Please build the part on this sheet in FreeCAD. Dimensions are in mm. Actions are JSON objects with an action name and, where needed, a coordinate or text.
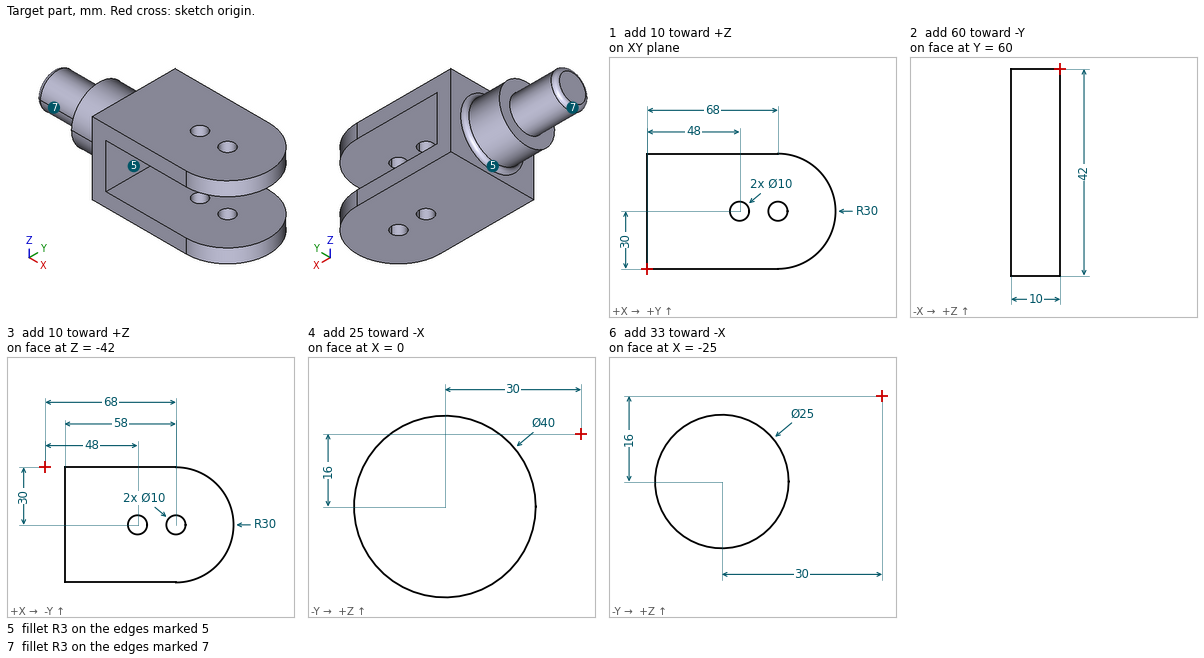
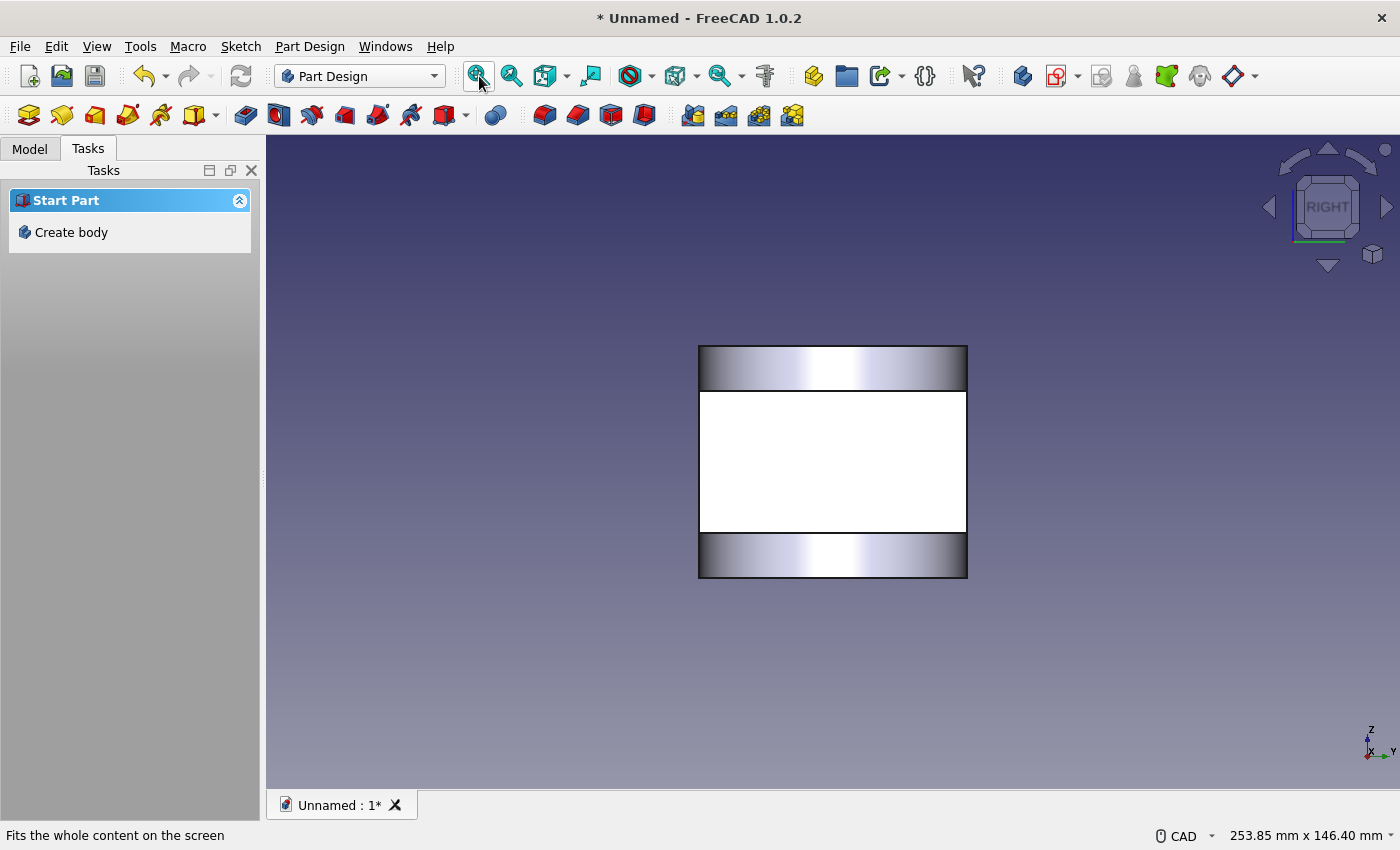
{"action": "key", "text": "5"}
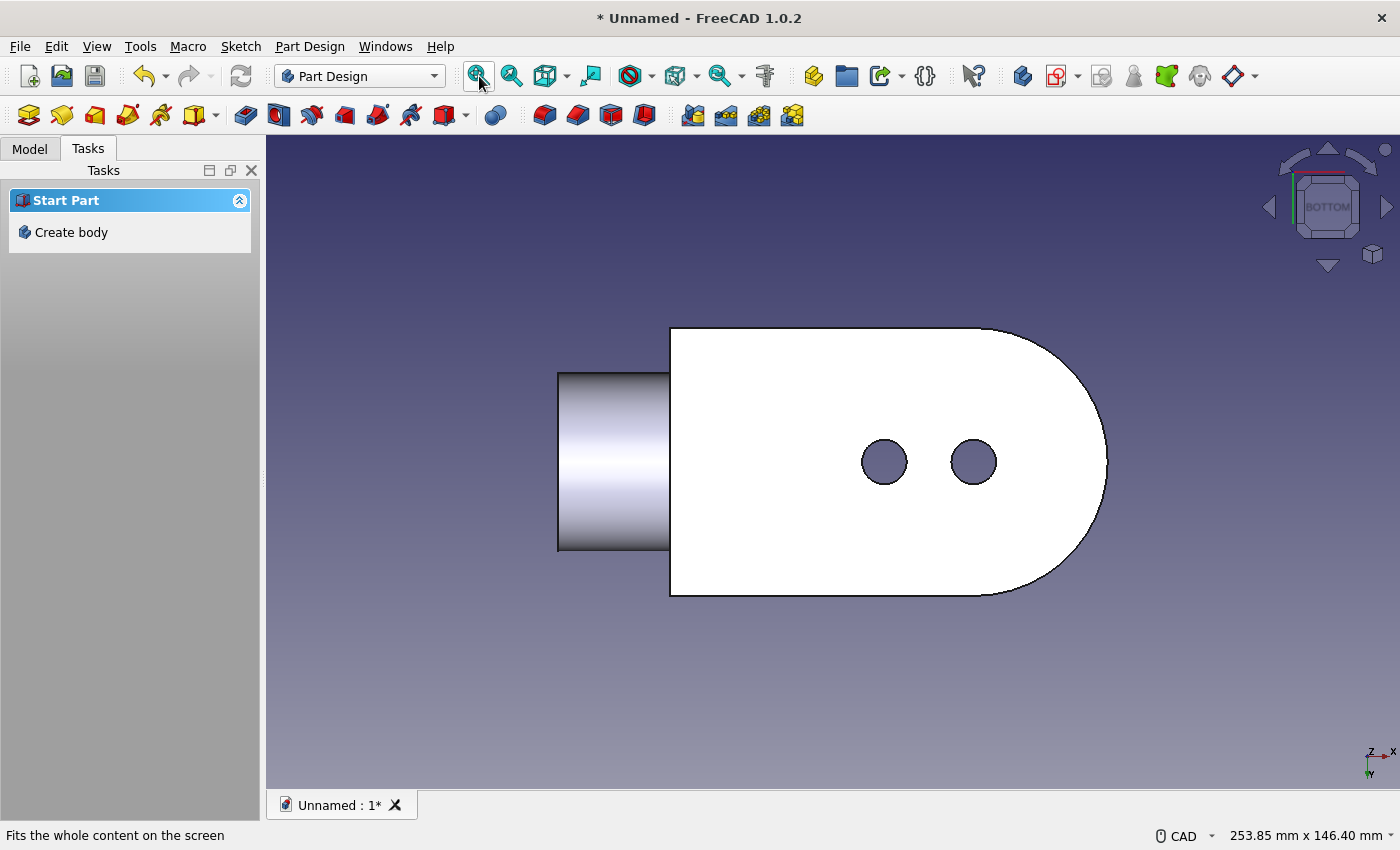
{"action": "key", "text": "4"}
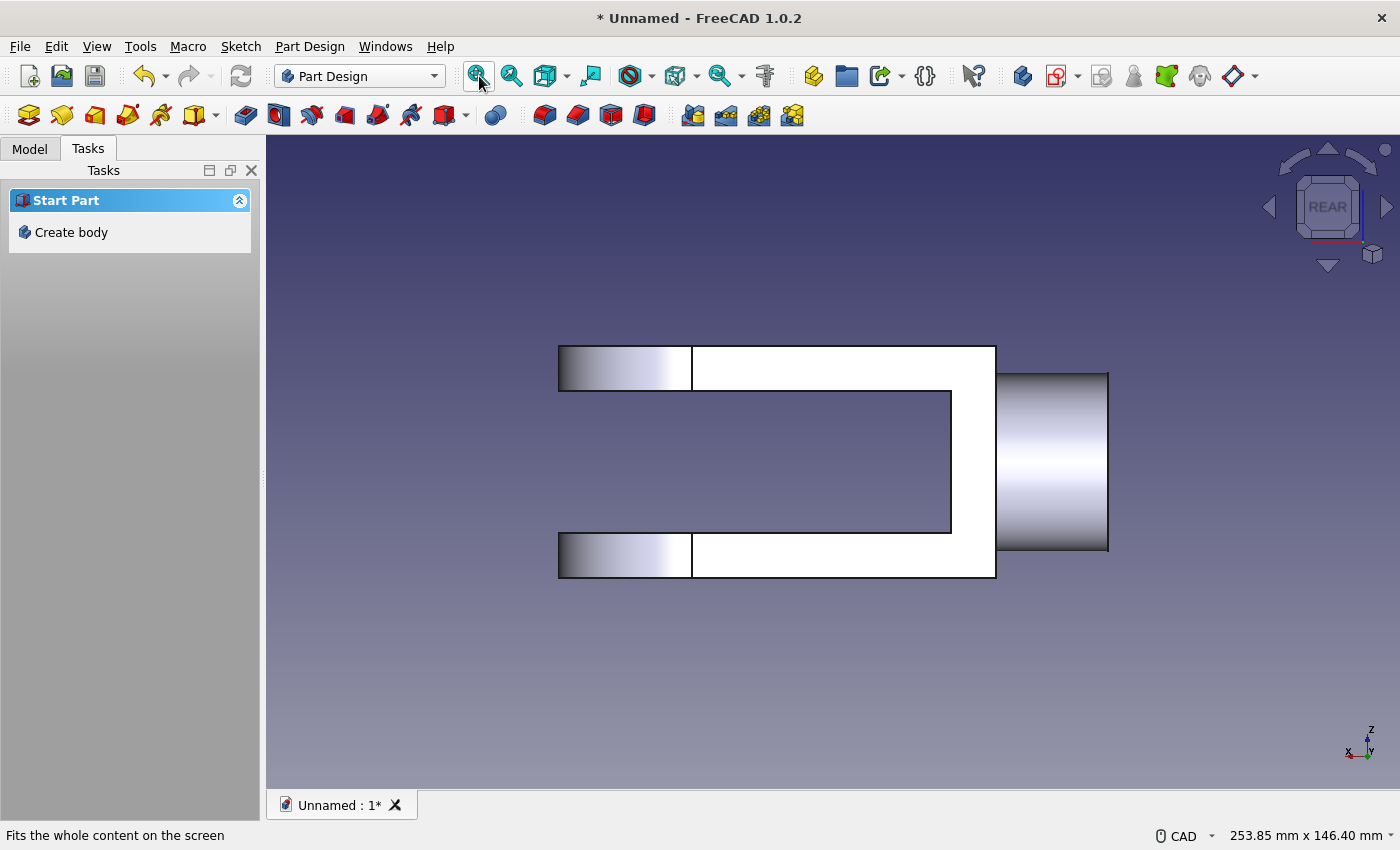
{"action": "key", "text": "6"}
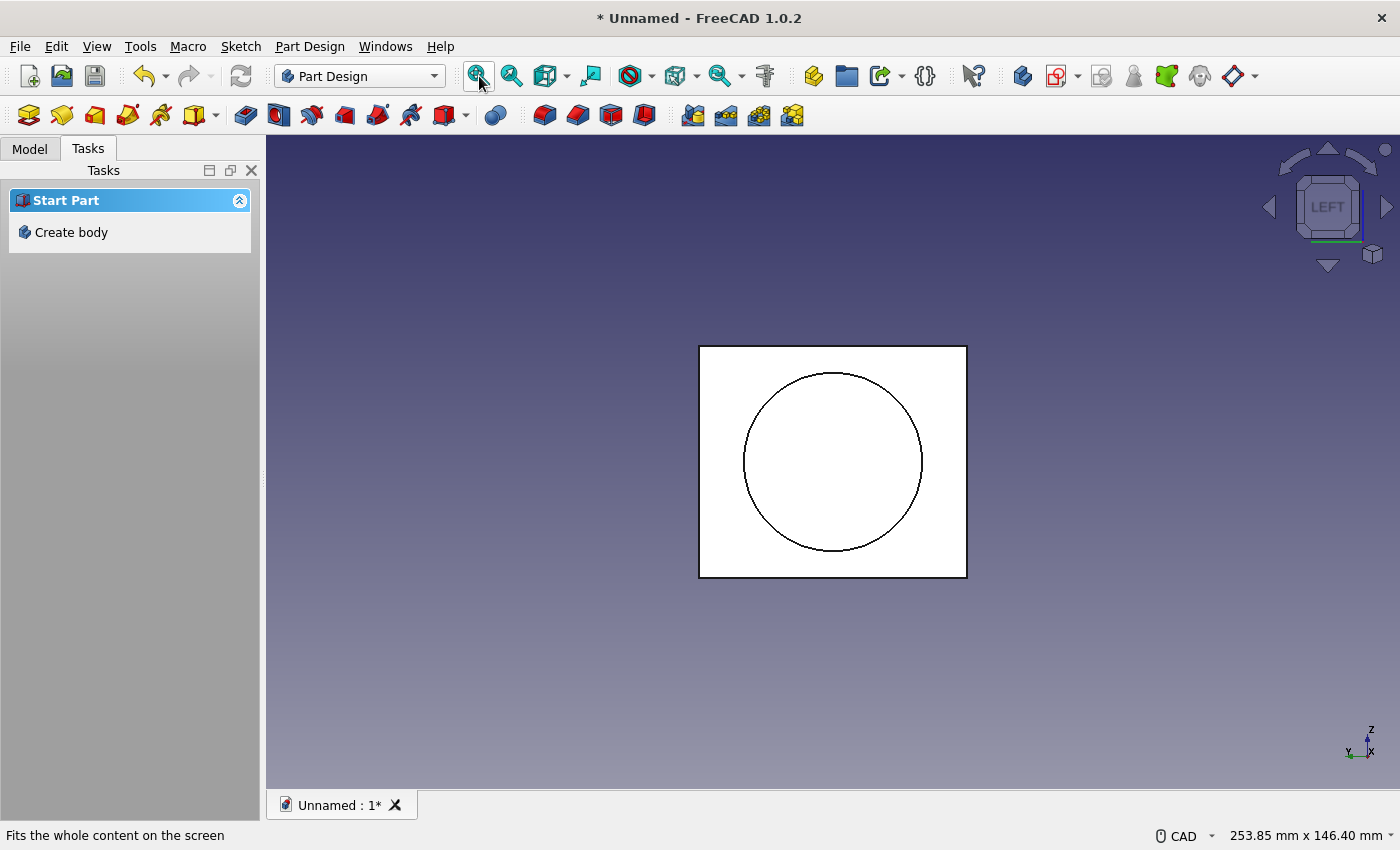
{"action": "key", "text": "v f"}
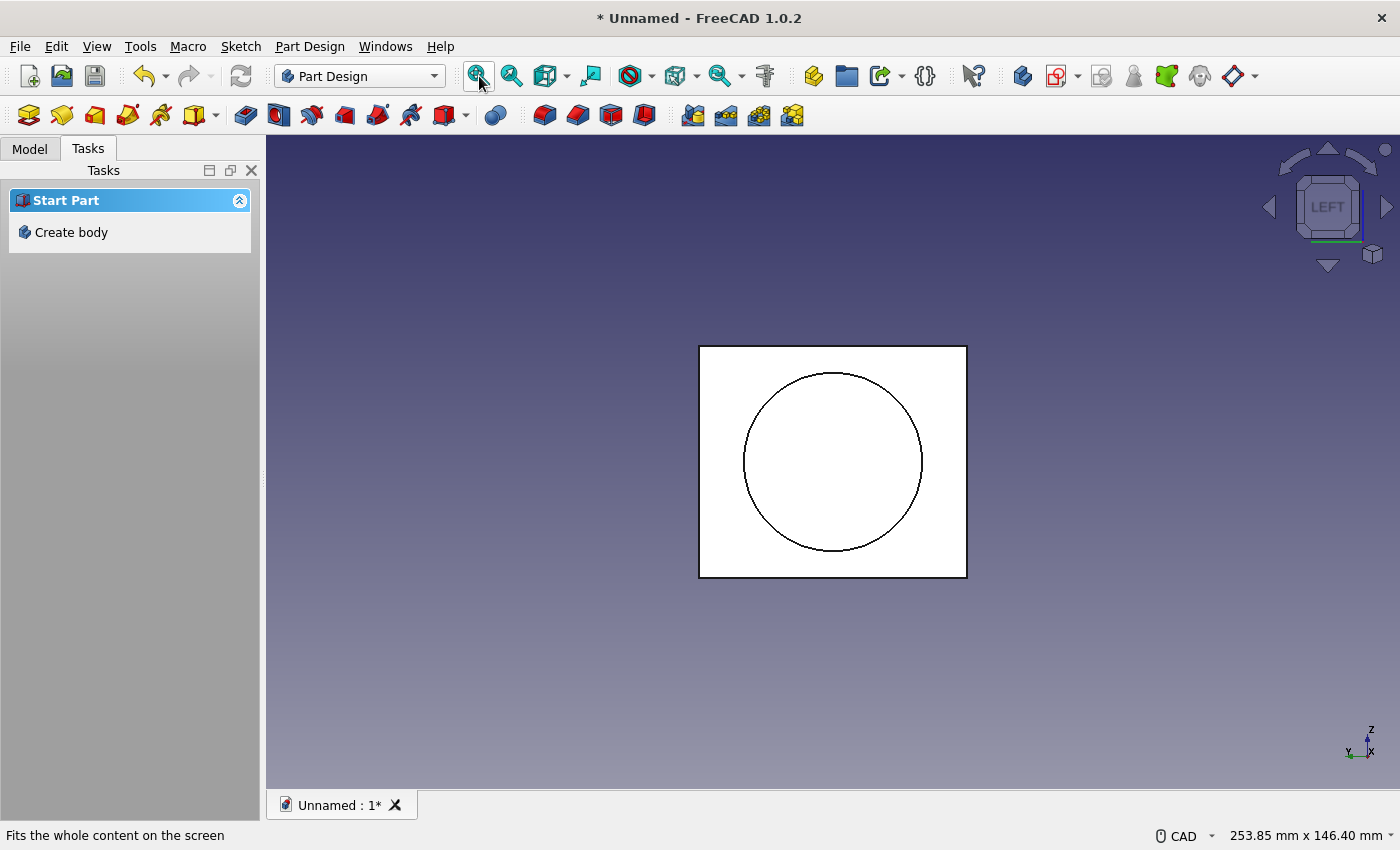
{"action": "key", "text": "v 3"}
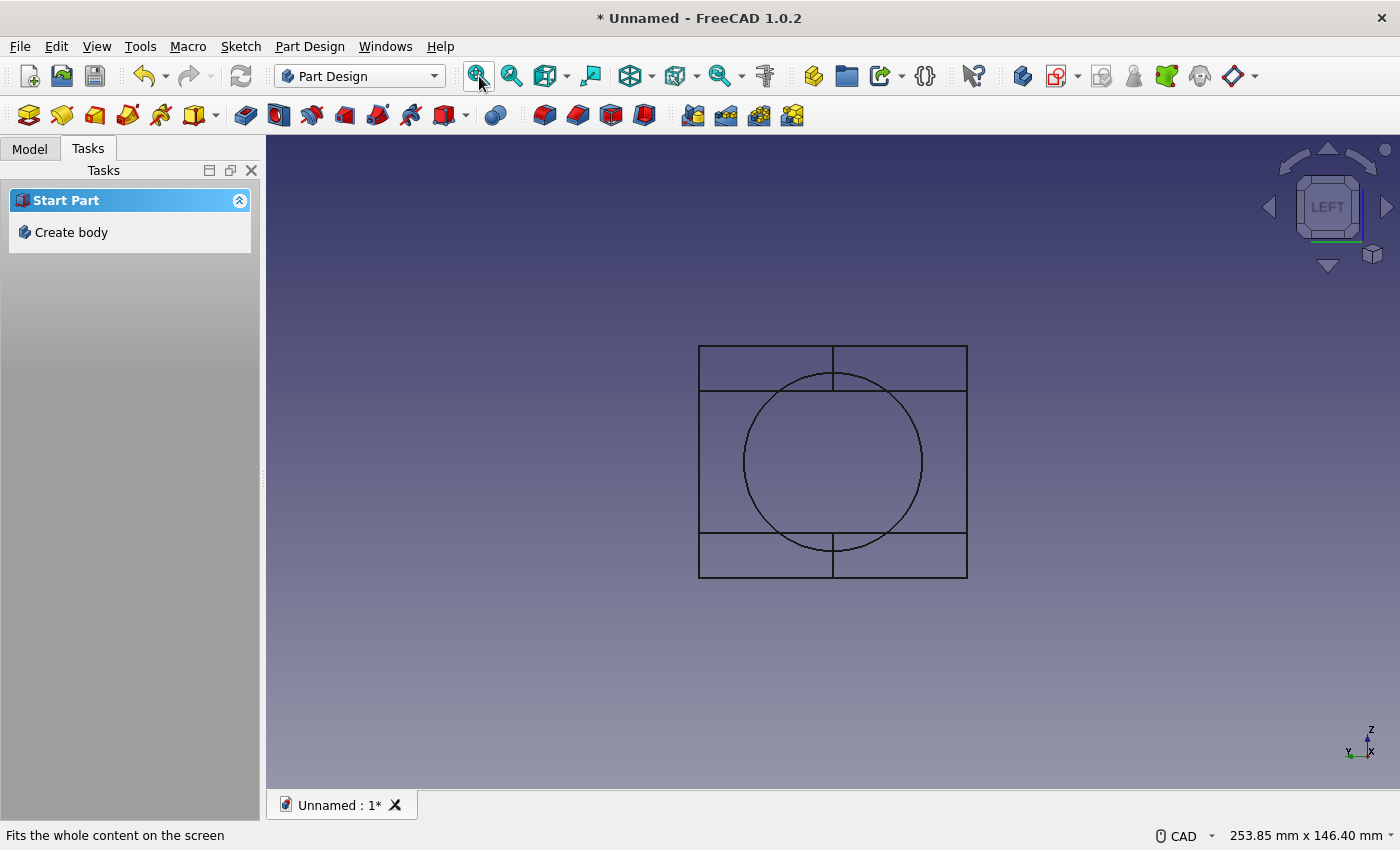
{"action": "key", "text": "0"}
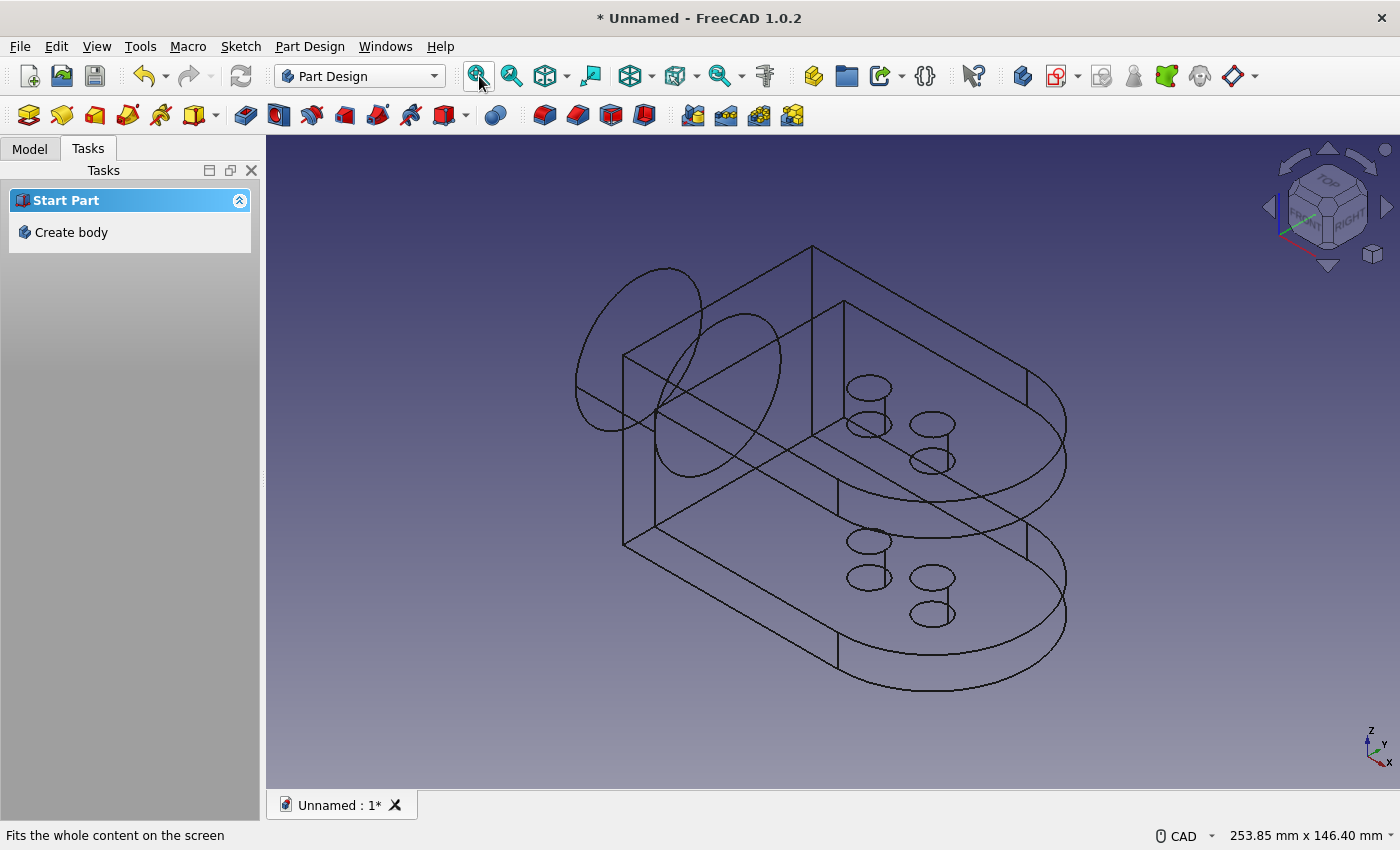
{"action": "left_click", "coordinate": [781, 358]}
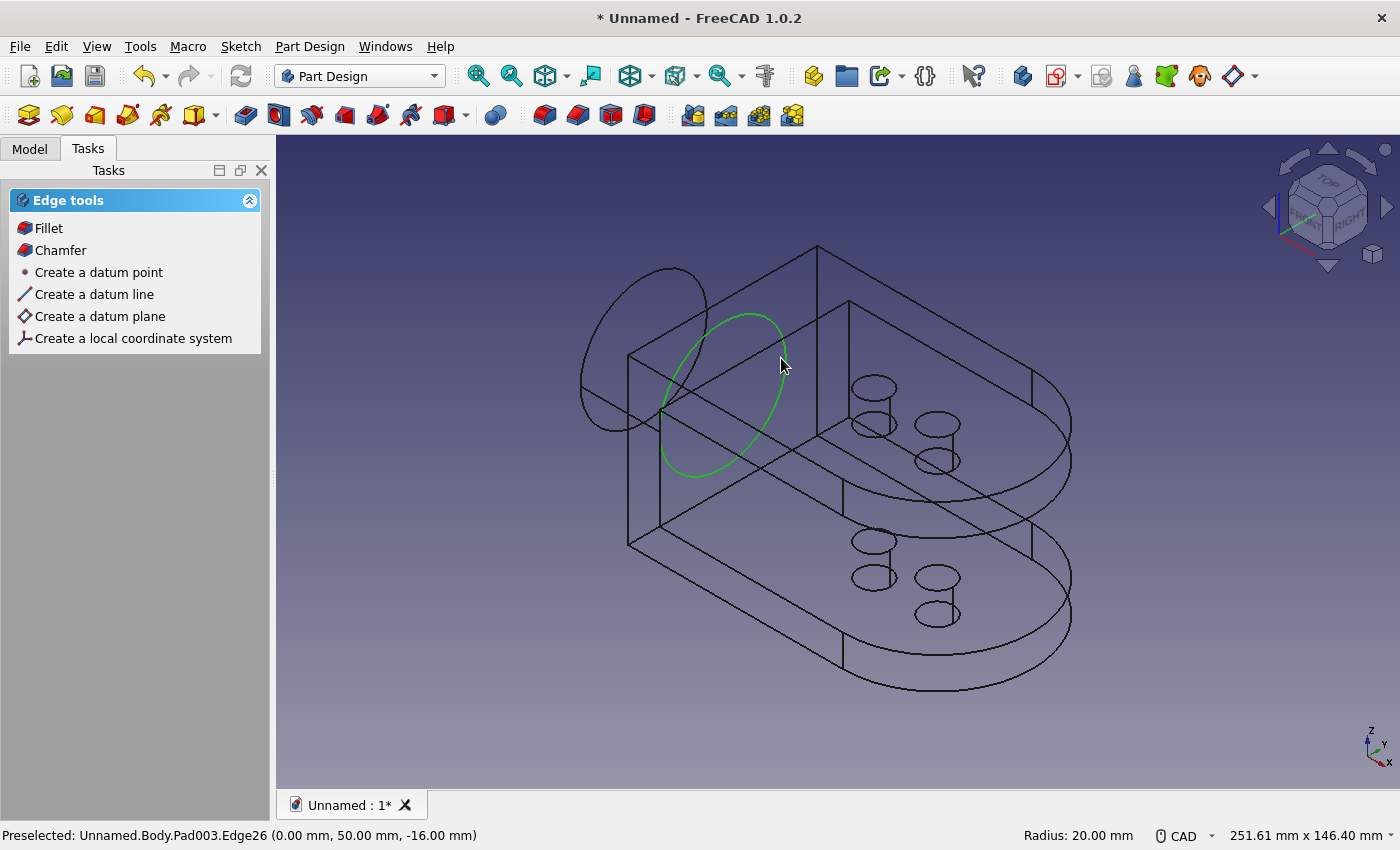
{"action": "key", "text": "v 1"}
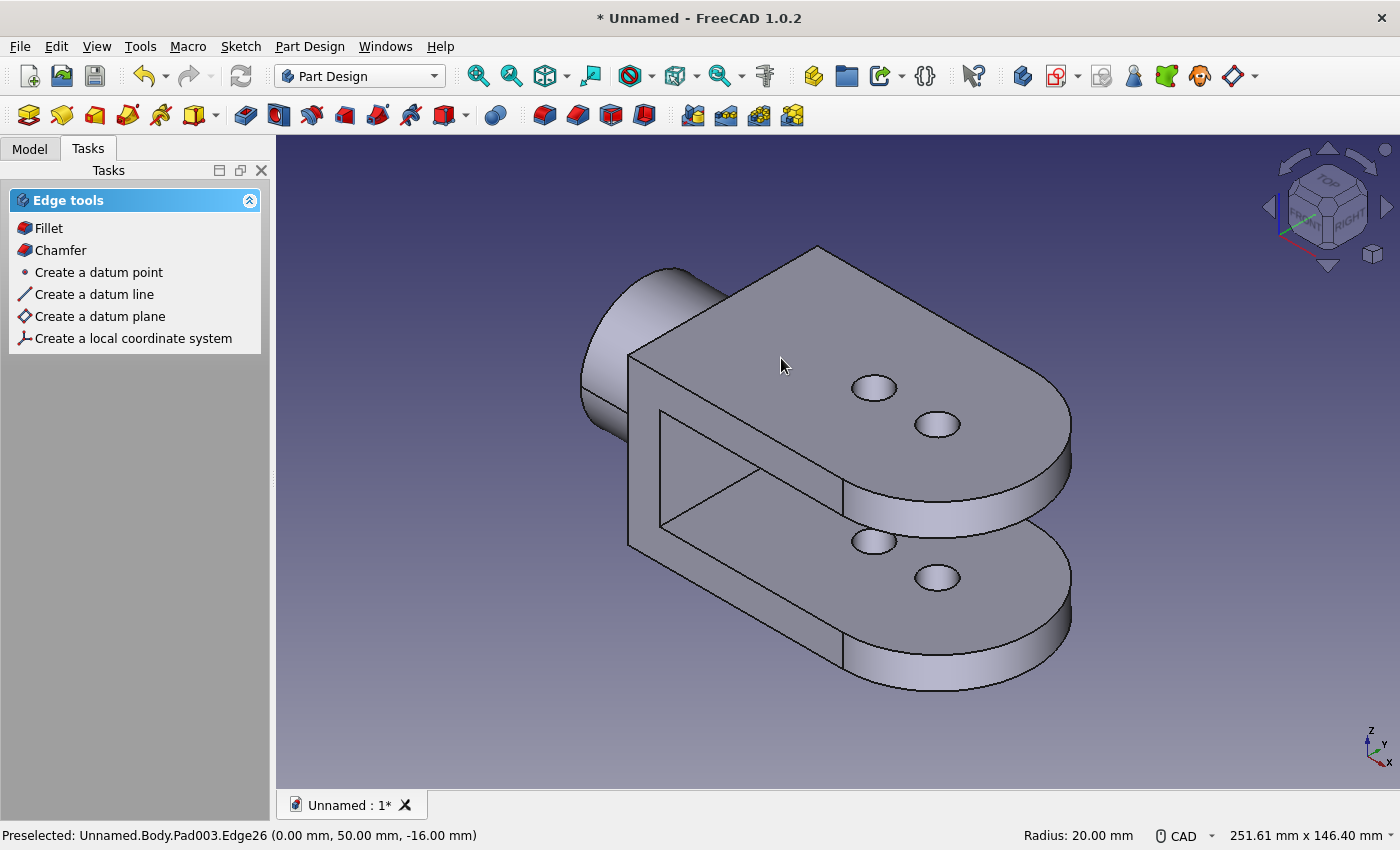
{"action": "left_click", "coordinate": [545, 116]}